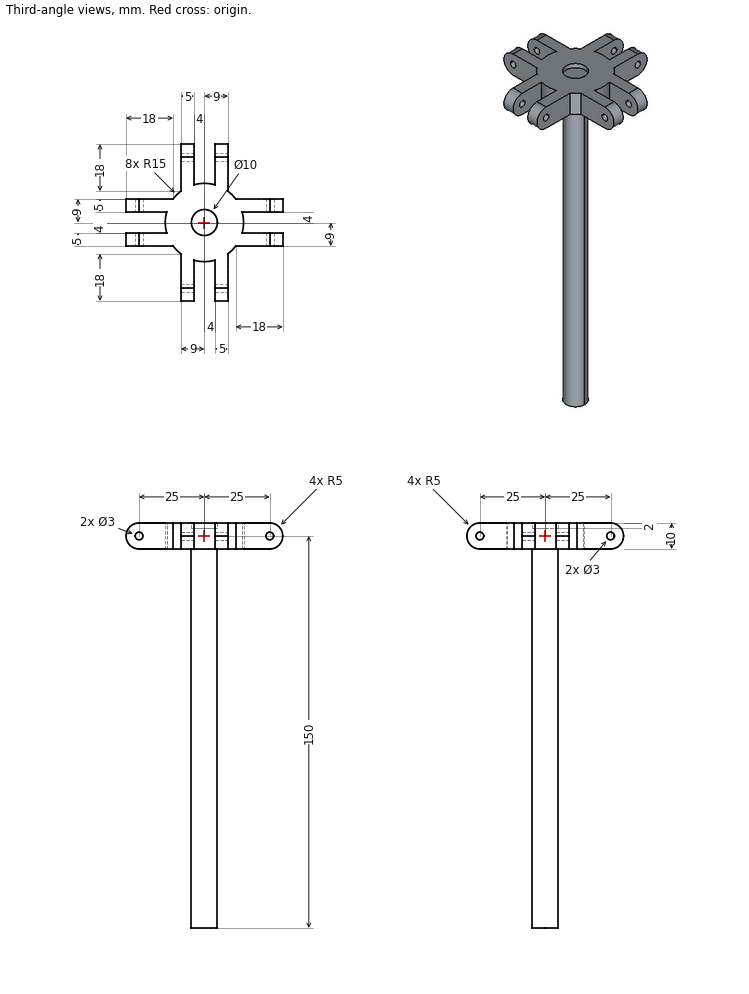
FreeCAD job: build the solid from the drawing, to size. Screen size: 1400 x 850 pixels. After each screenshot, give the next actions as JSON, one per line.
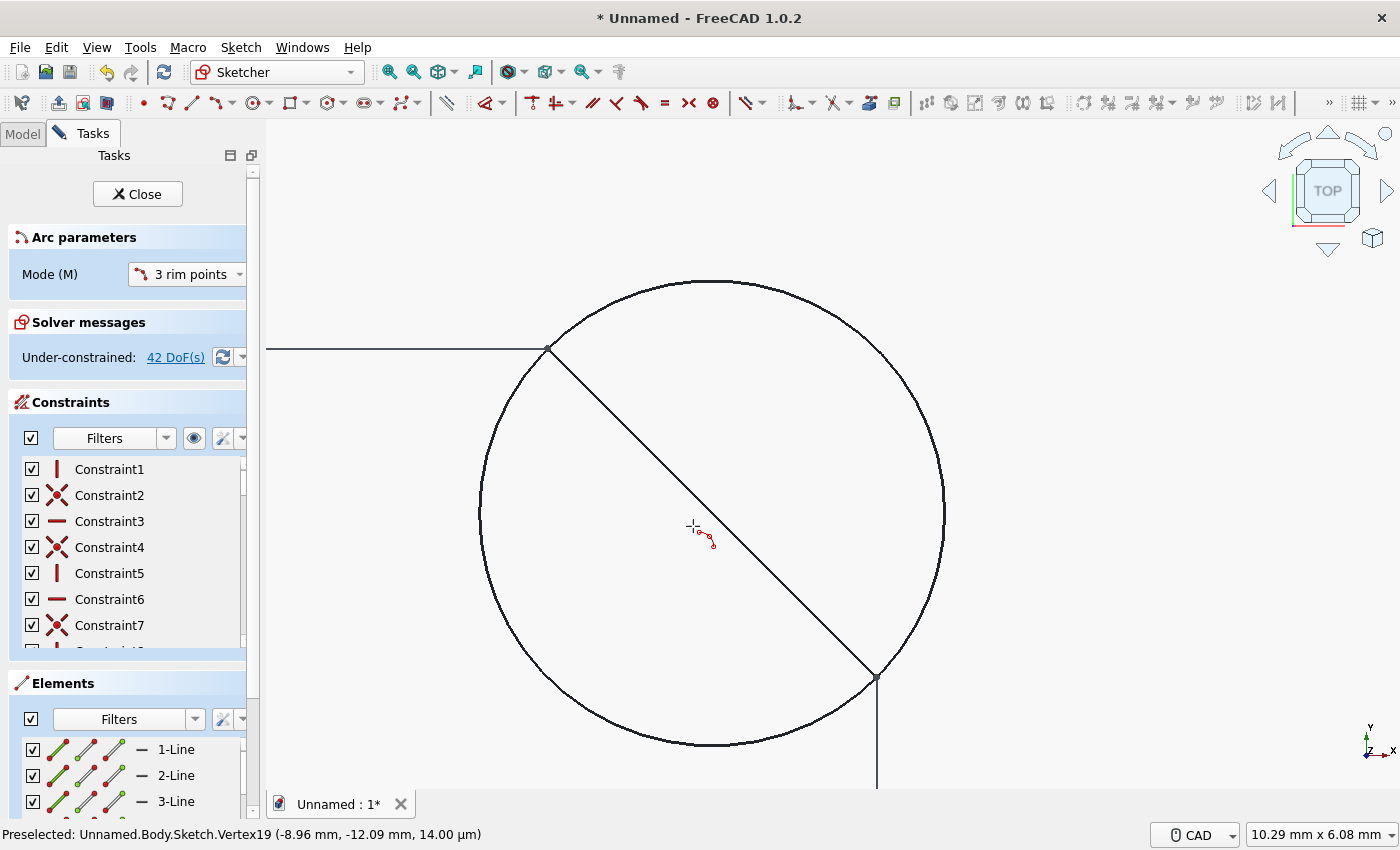
{"action": "left_click", "coordinate": [695, 514]}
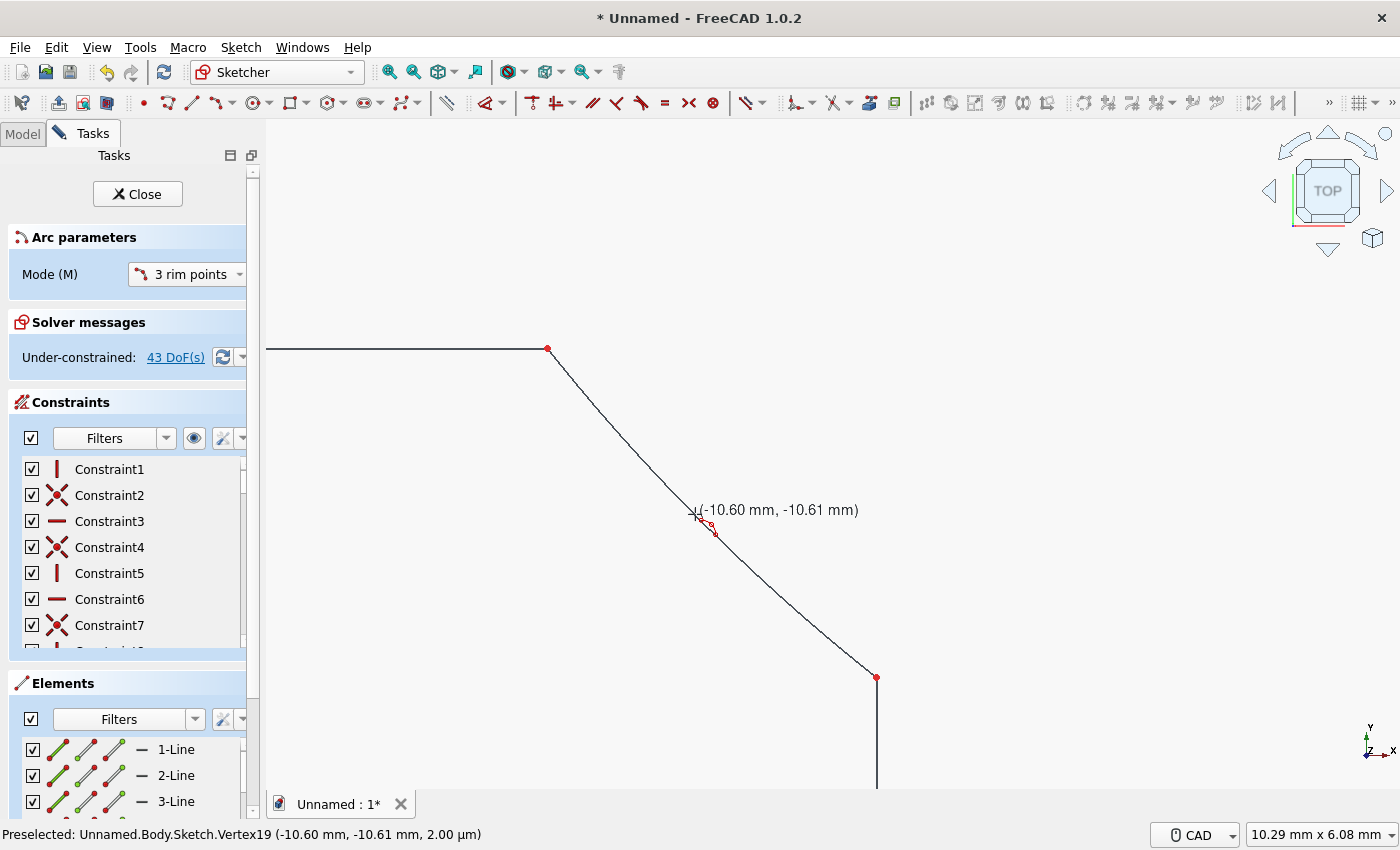
{"action": "scroll", "coordinate": [693, 526], "scroll_direction": "down", "scroll_amount": 14}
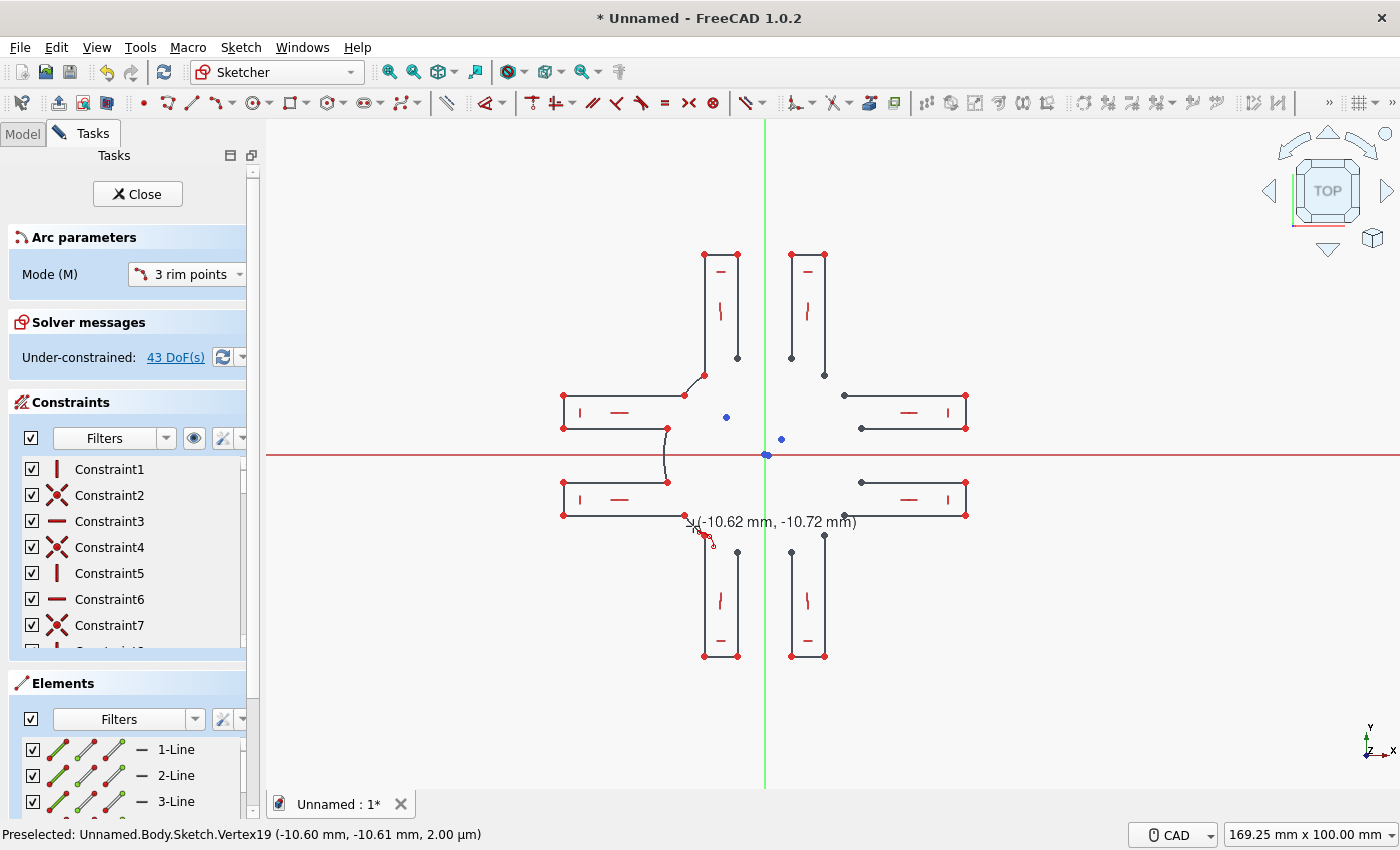
{"action": "left_click", "coordinate": [738, 553]}
{"action": "left_click", "coordinate": [792, 553]}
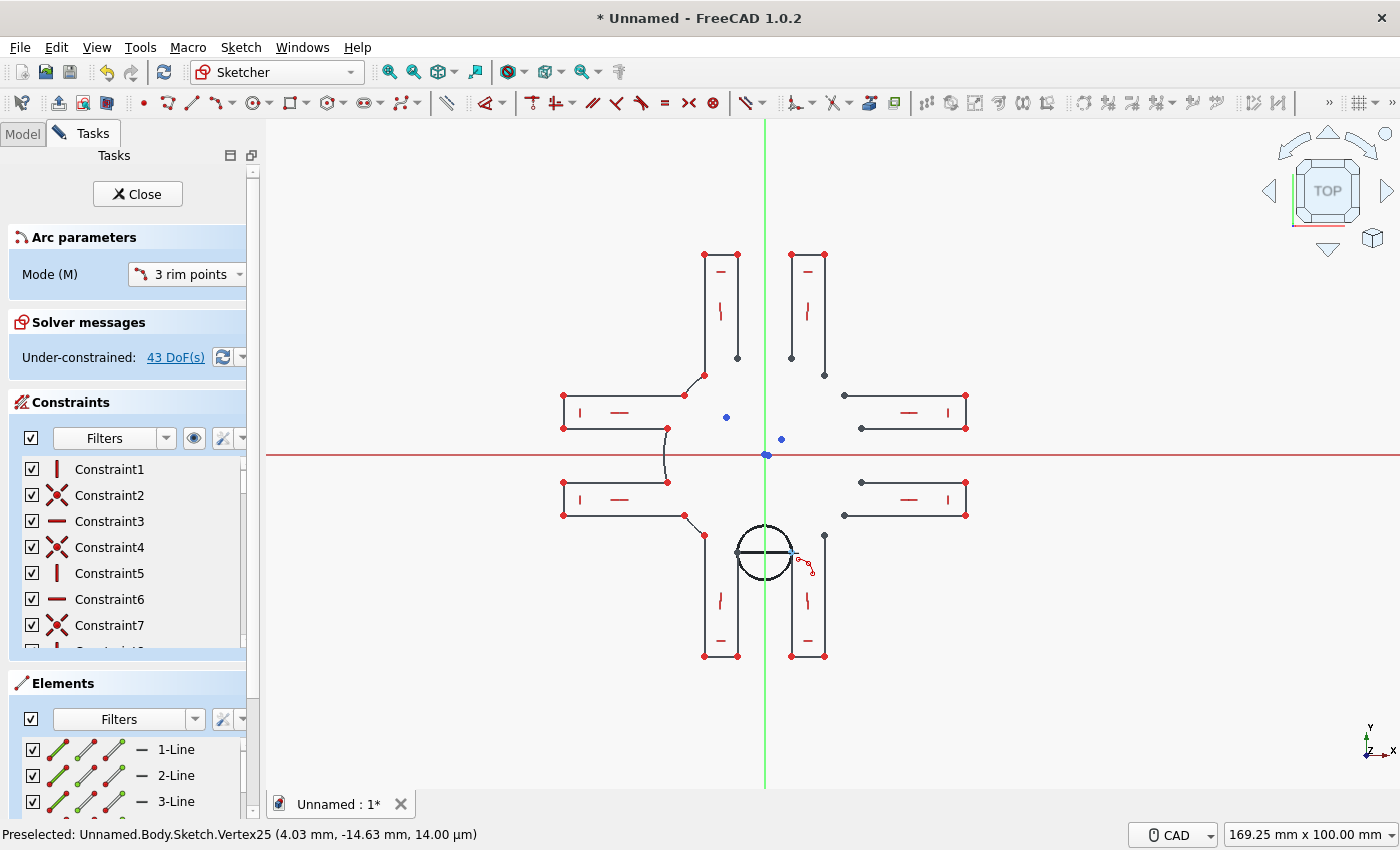
{"action": "scroll", "coordinate": [759, 555], "scroll_direction": "up", "scroll_amount": 8}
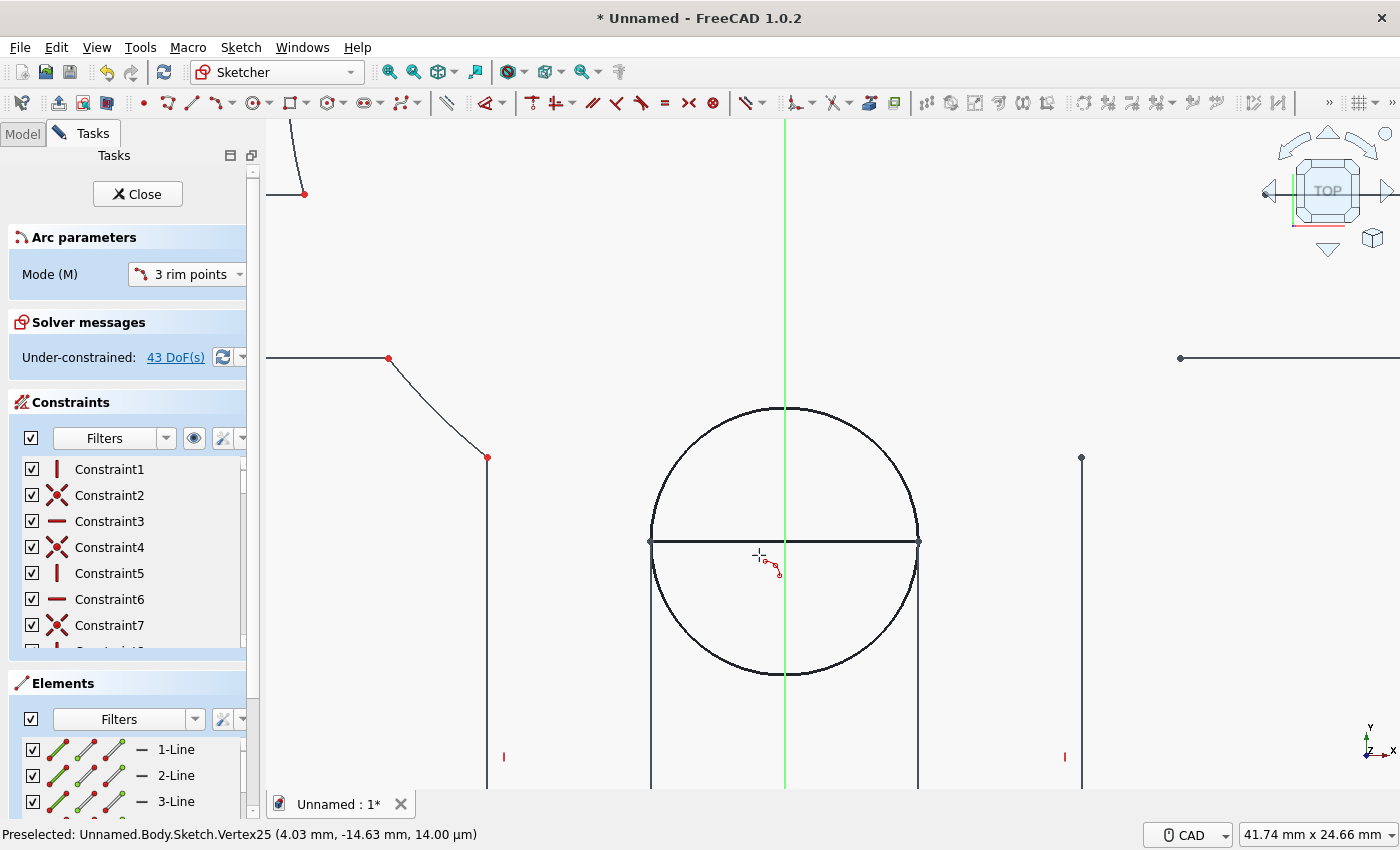
{"action": "left_click", "coordinate": [758, 553]}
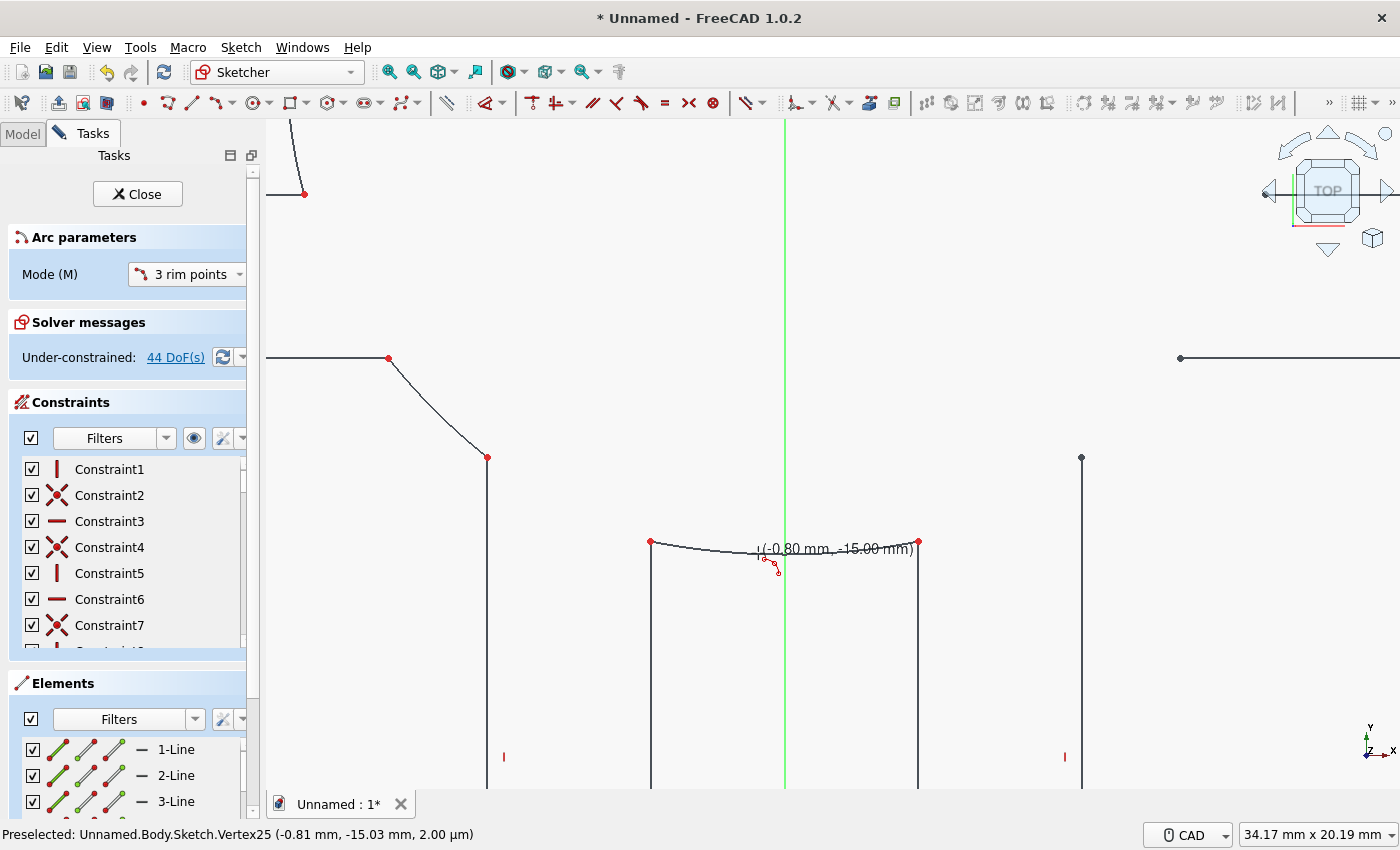
{"action": "scroll", "coordinate": [759, 555], "scroll_direction": "down", "scroll_amount": 8}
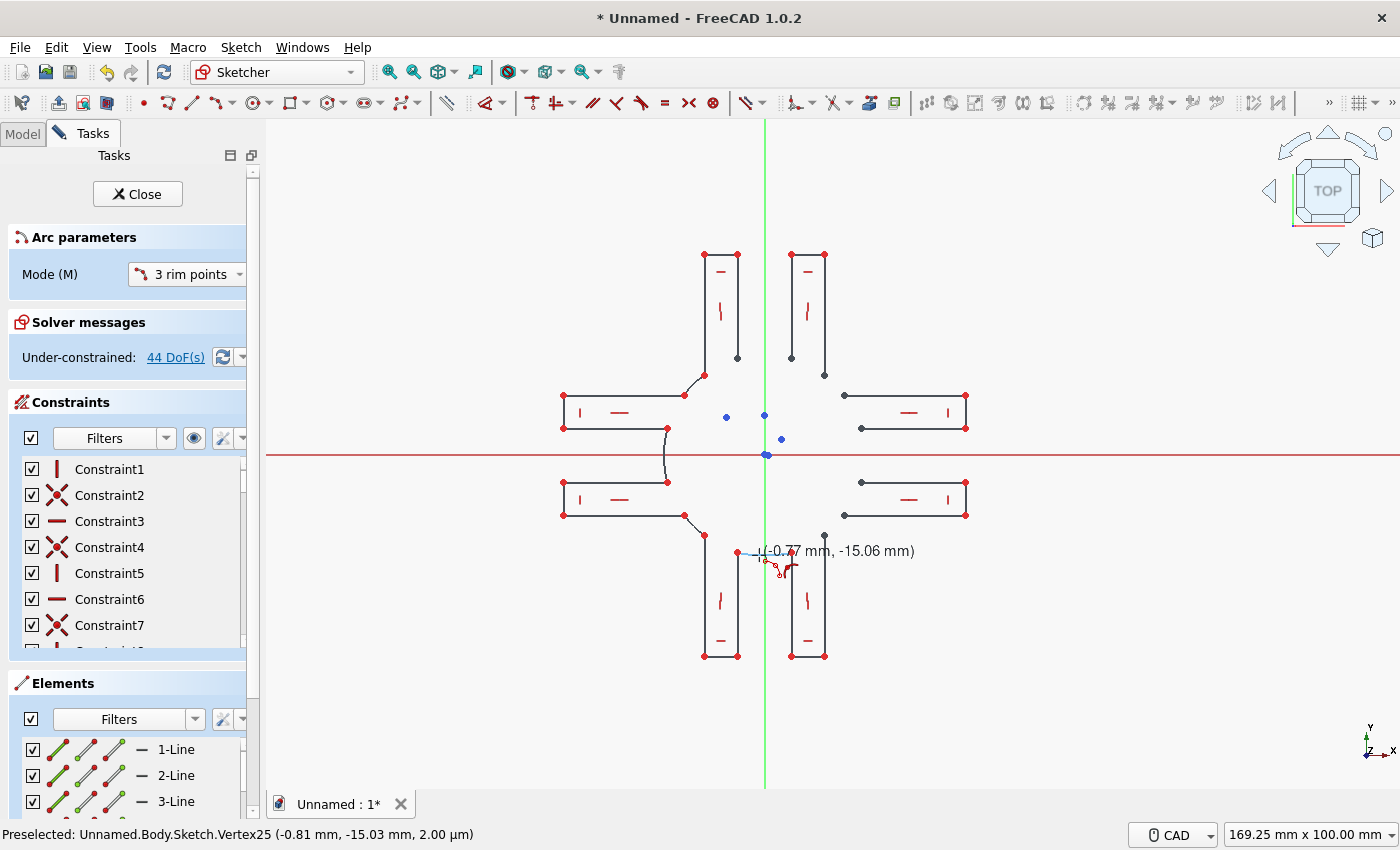
{"action": "left_click", "coordinate": [825, 536]}
{"action": "left_click", "coordinate": [845, 516]}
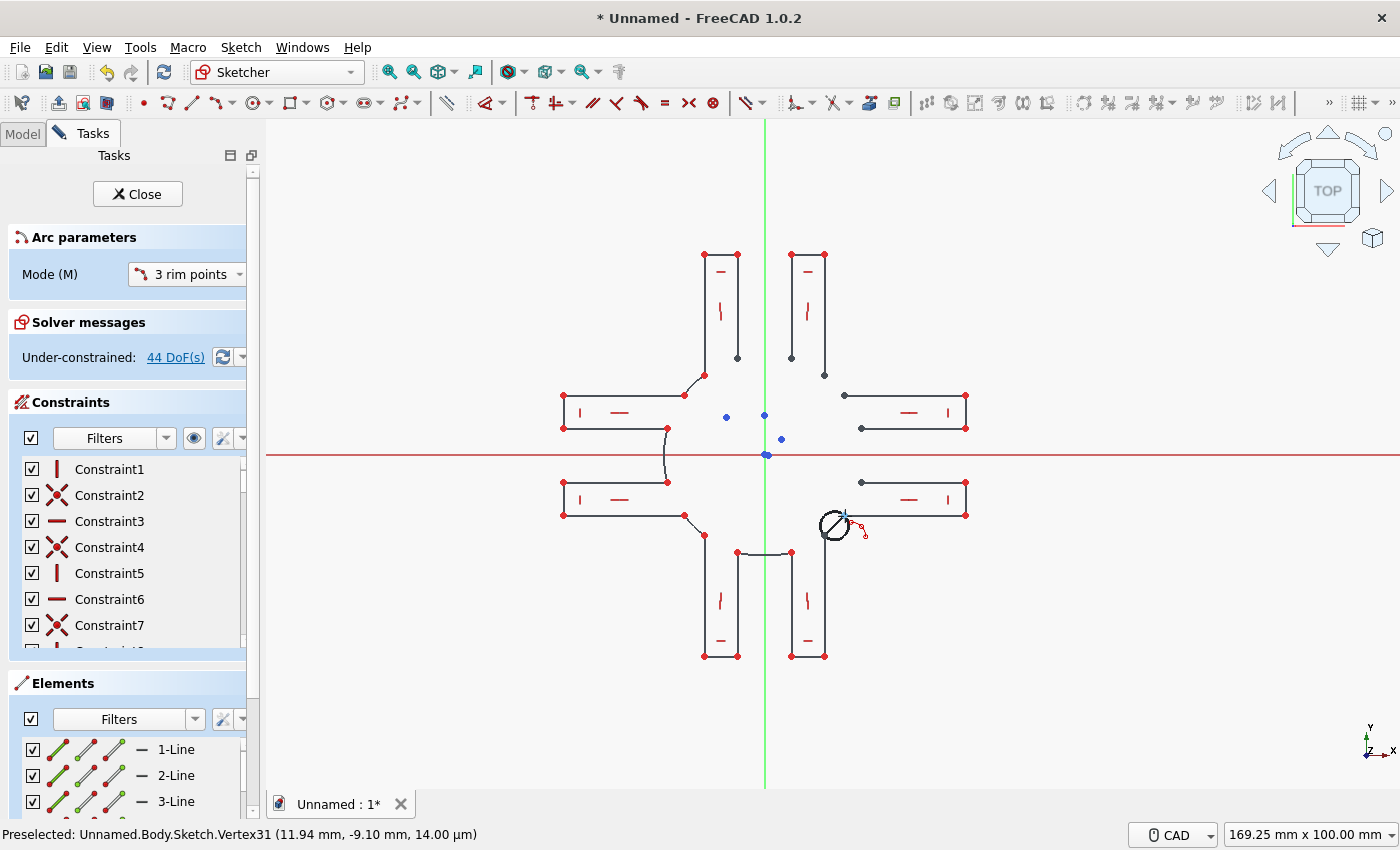
{"action": "scroll", "coordinate": [836, 526], "scroll_direction": "up", "scroll_amount": 14}